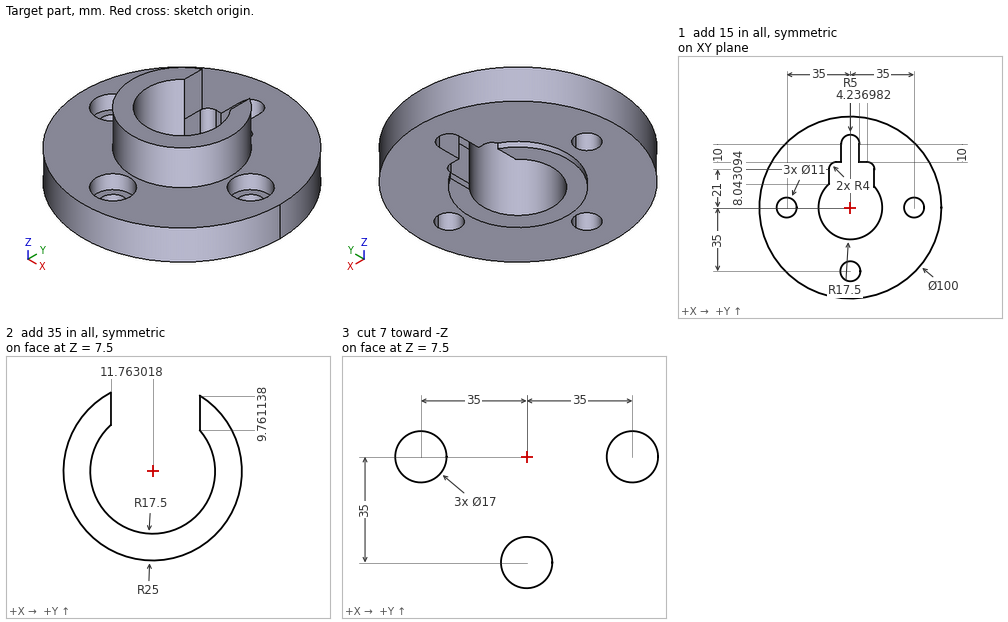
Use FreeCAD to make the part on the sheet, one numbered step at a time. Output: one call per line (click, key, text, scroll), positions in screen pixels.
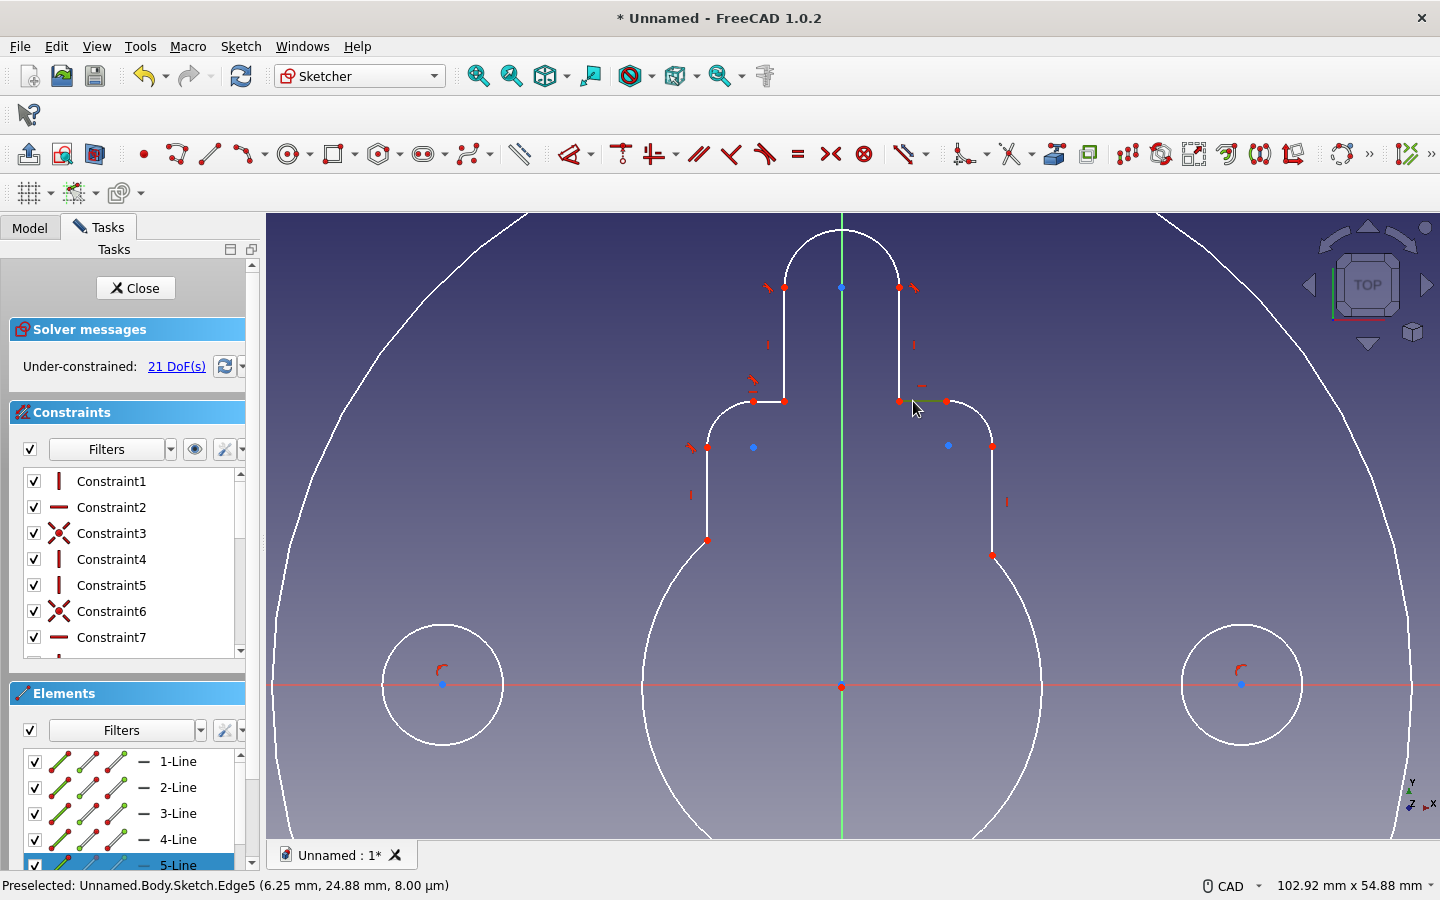
click(988, 426)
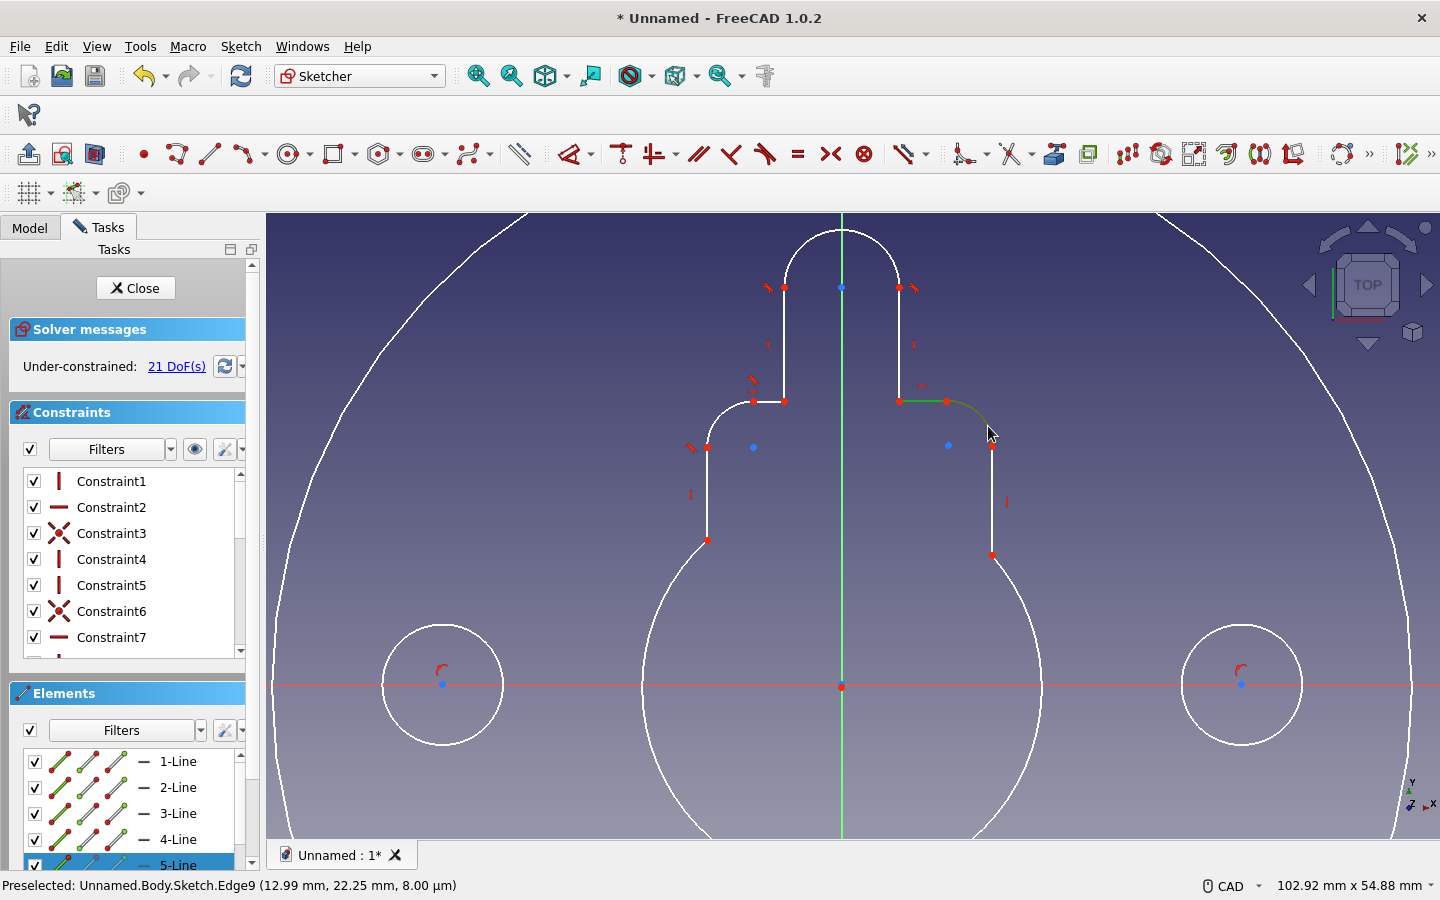
key(t)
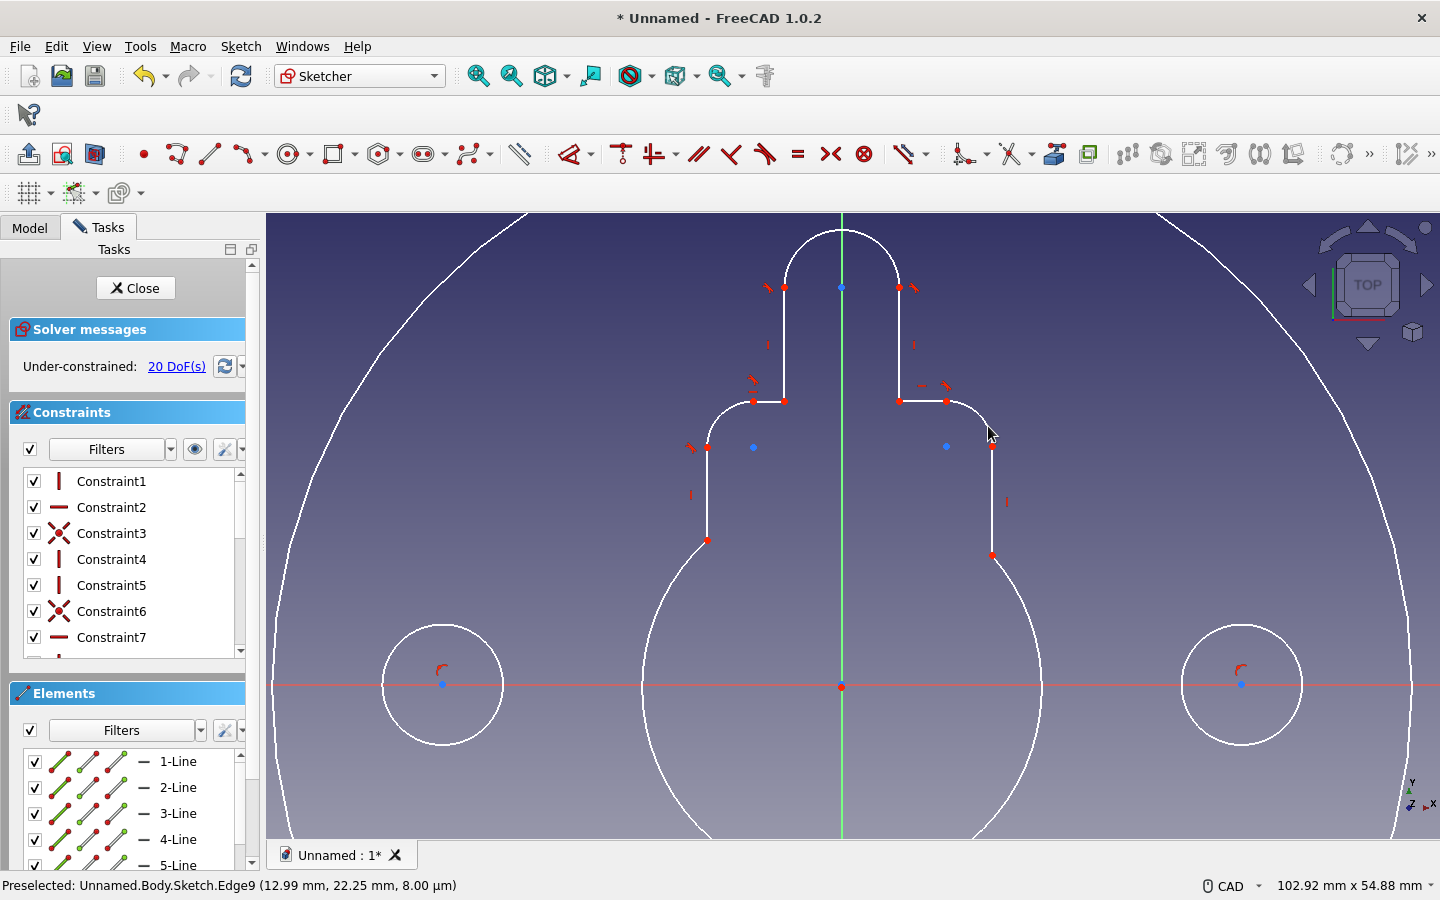
click(992, 479)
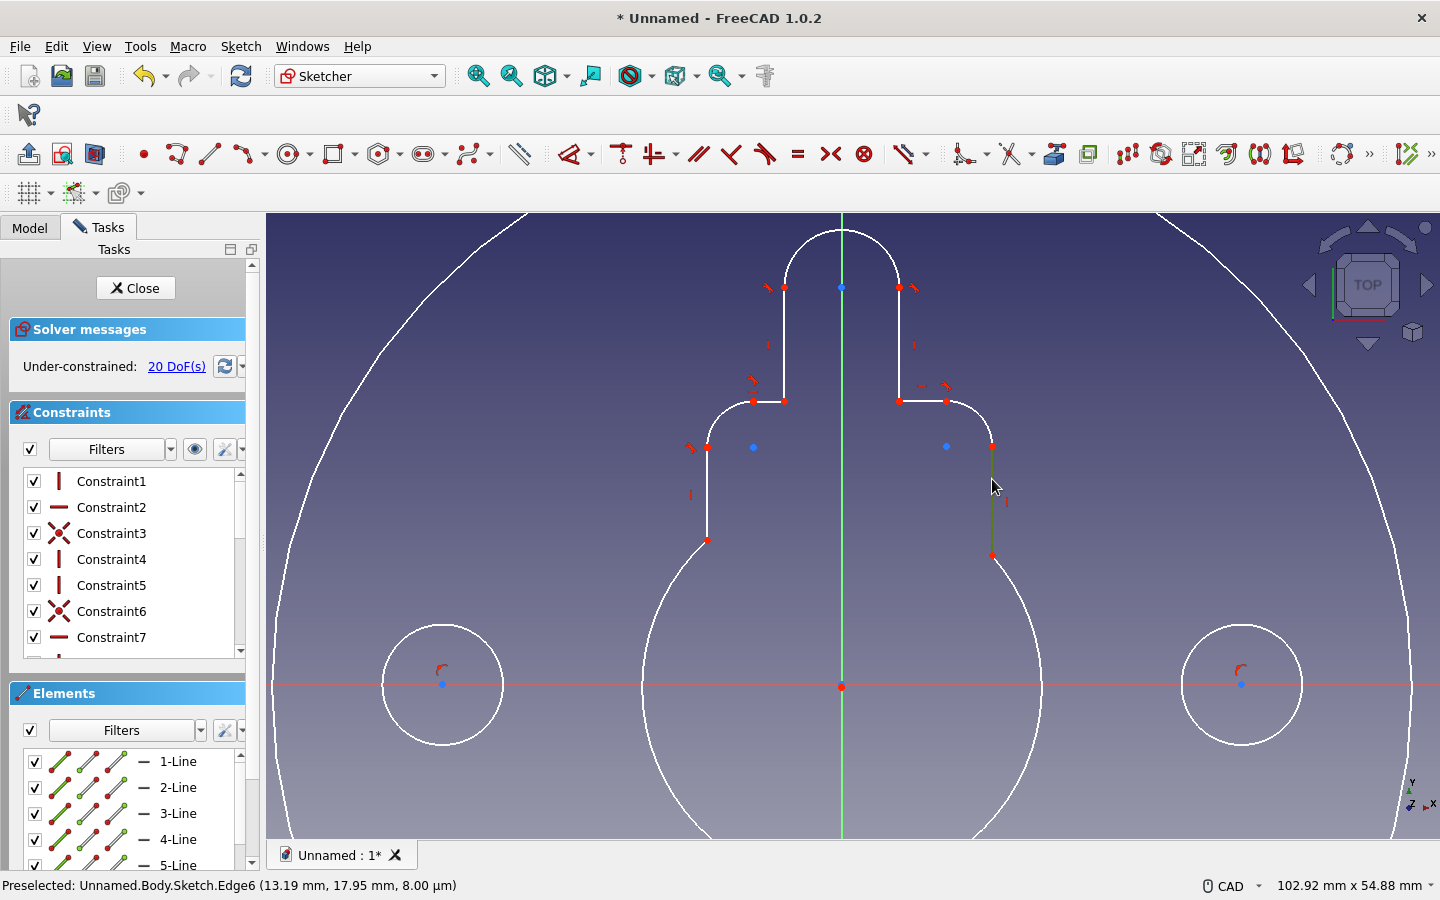
click(987, 426)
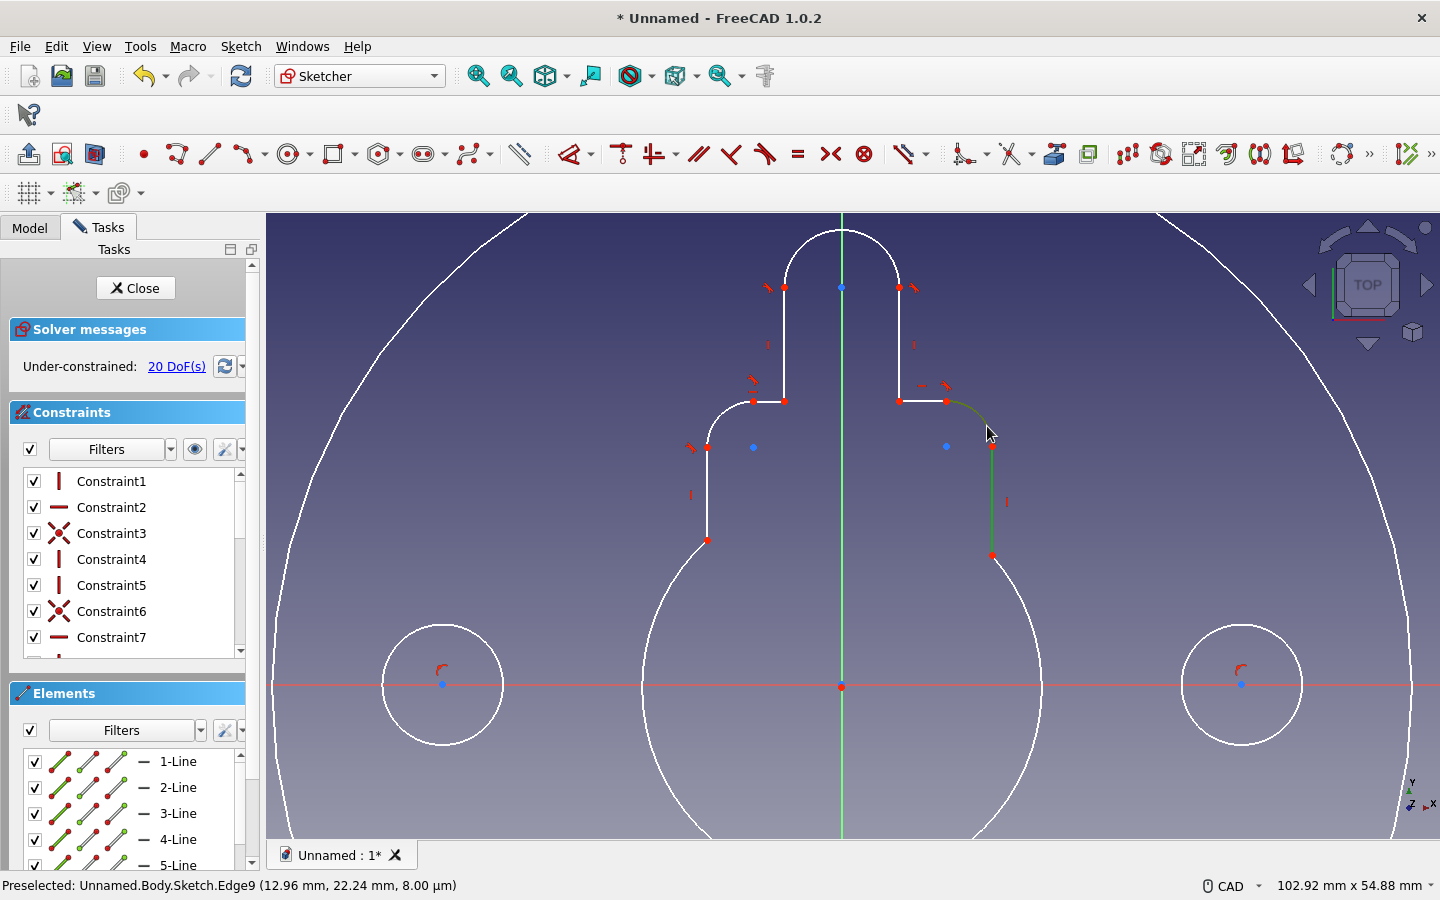
click(765, 154)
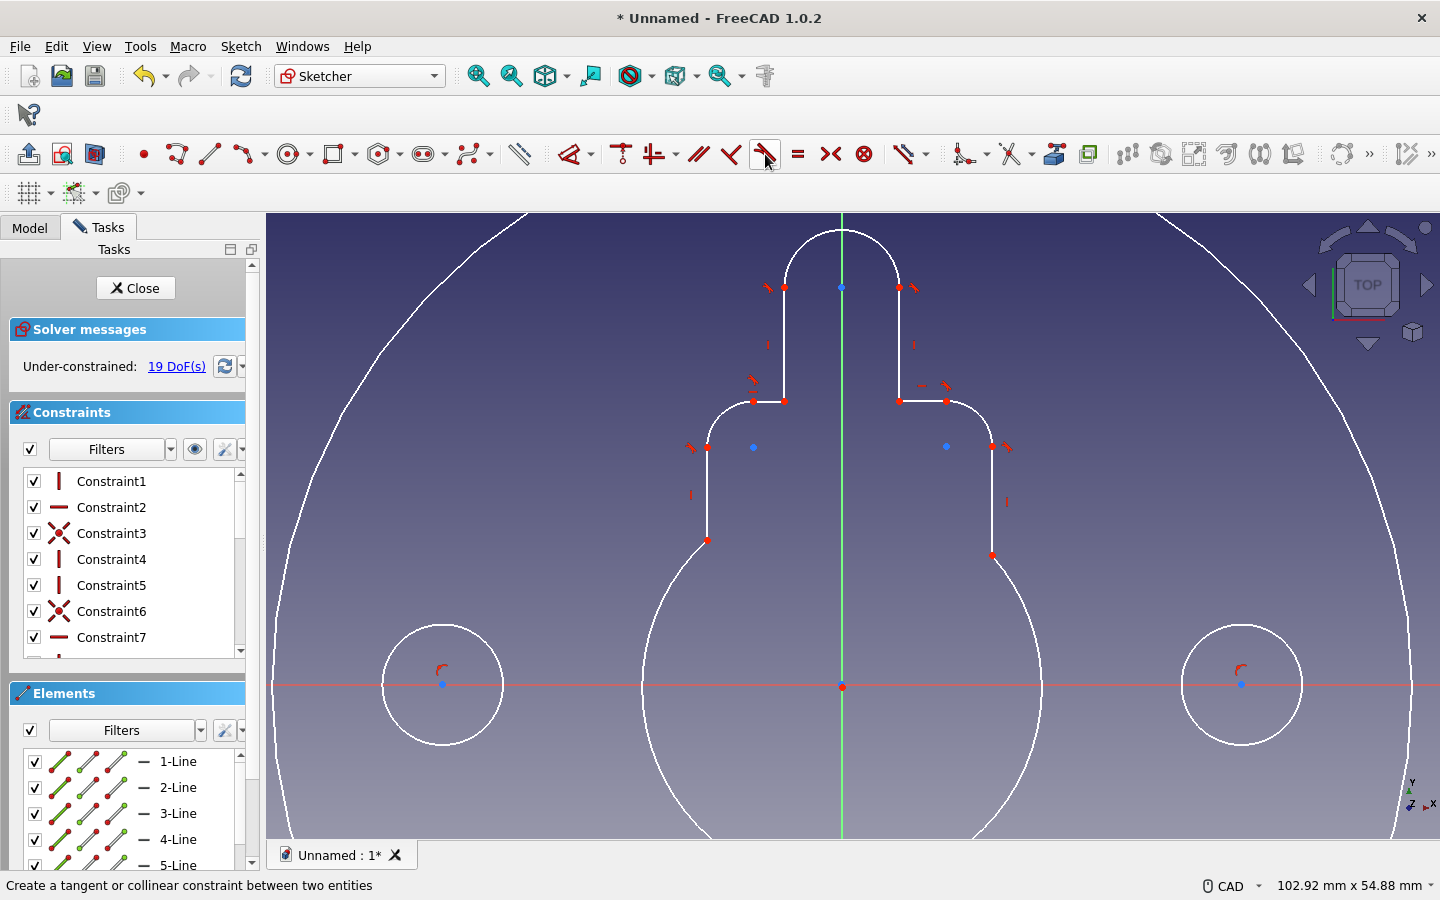
drag(832, 675, 852, 698)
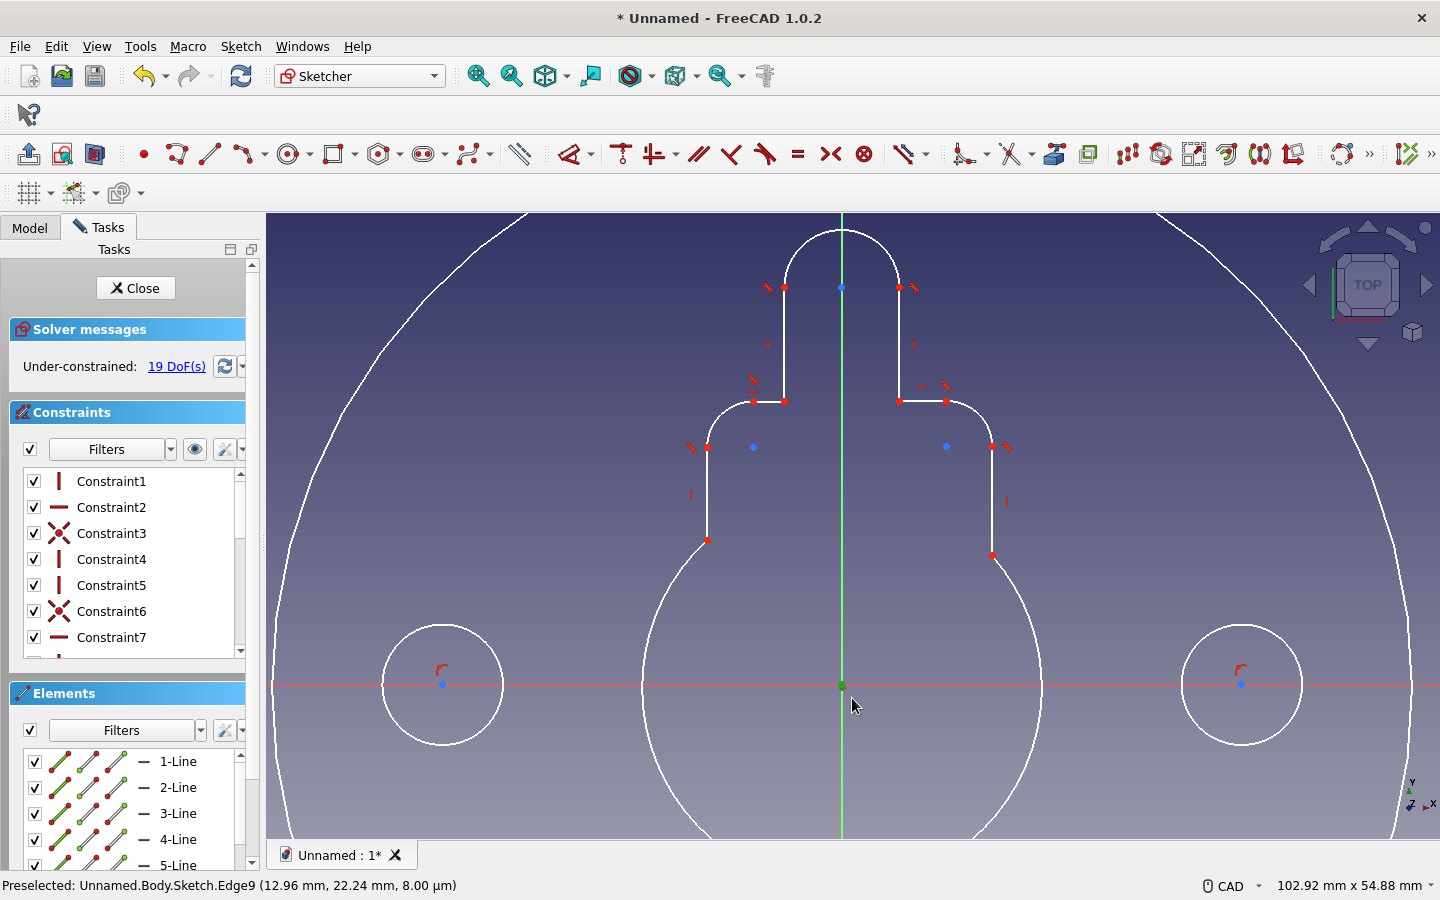
key(c)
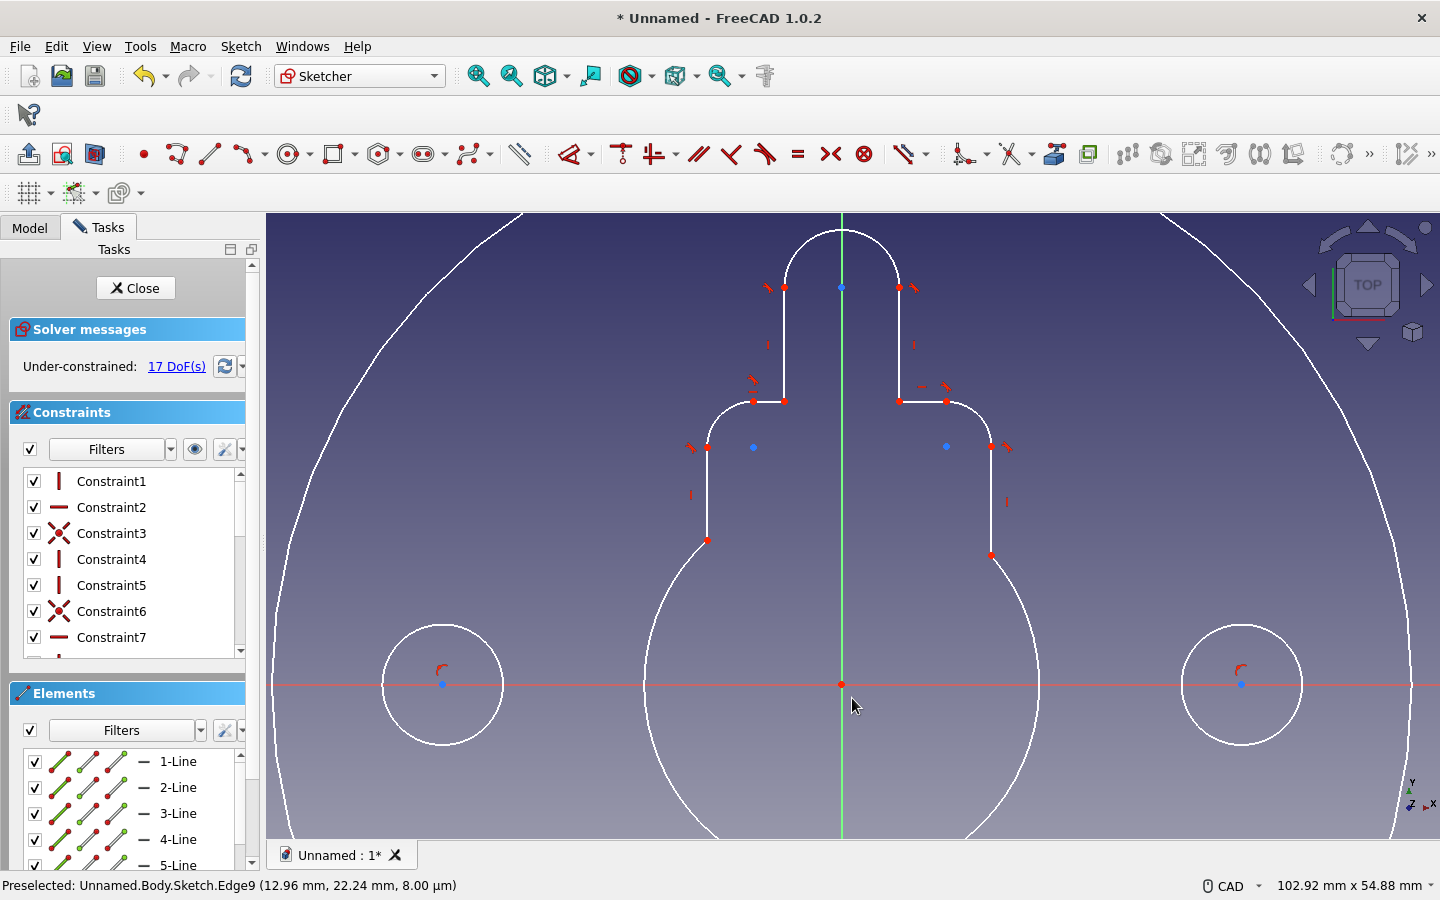
click(732, 407)